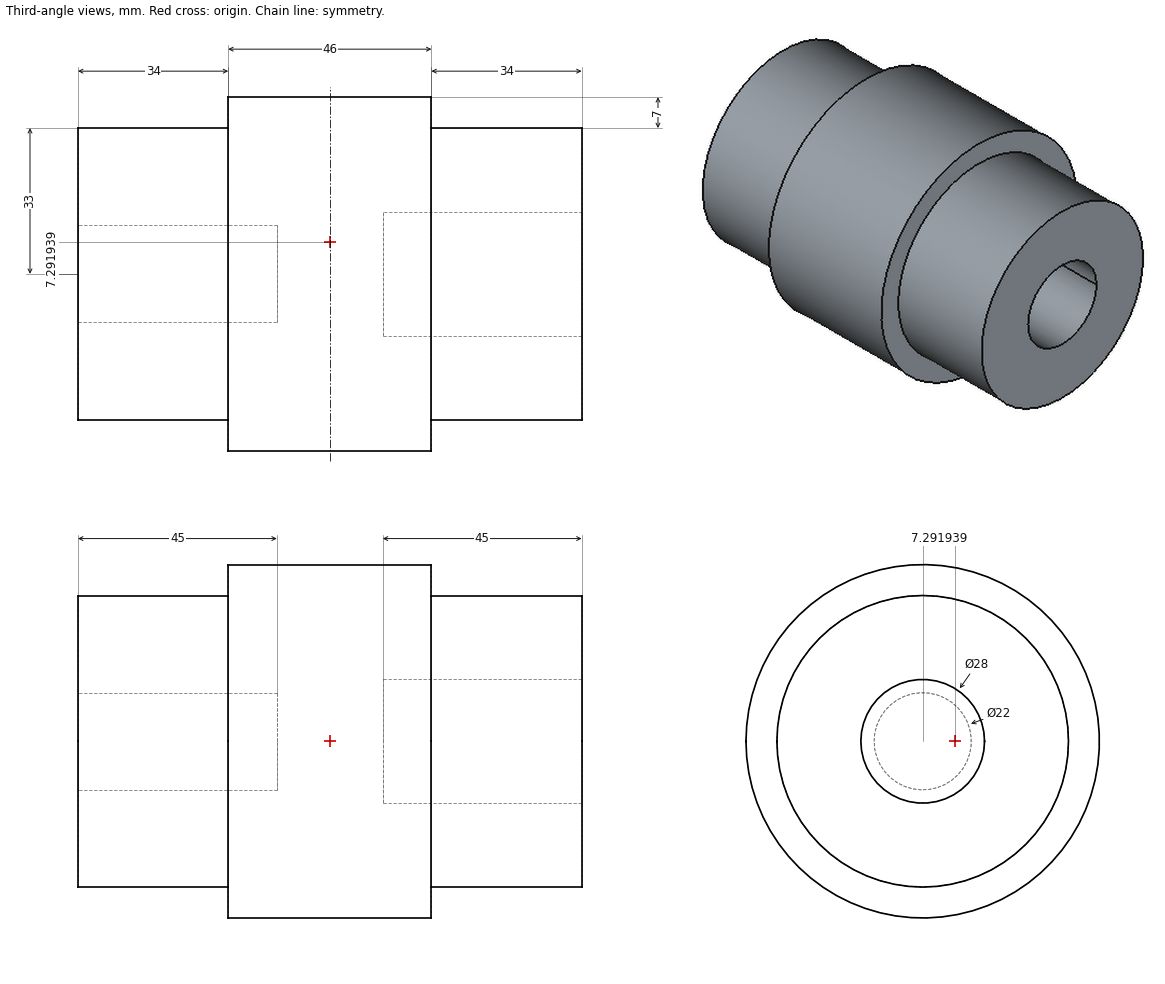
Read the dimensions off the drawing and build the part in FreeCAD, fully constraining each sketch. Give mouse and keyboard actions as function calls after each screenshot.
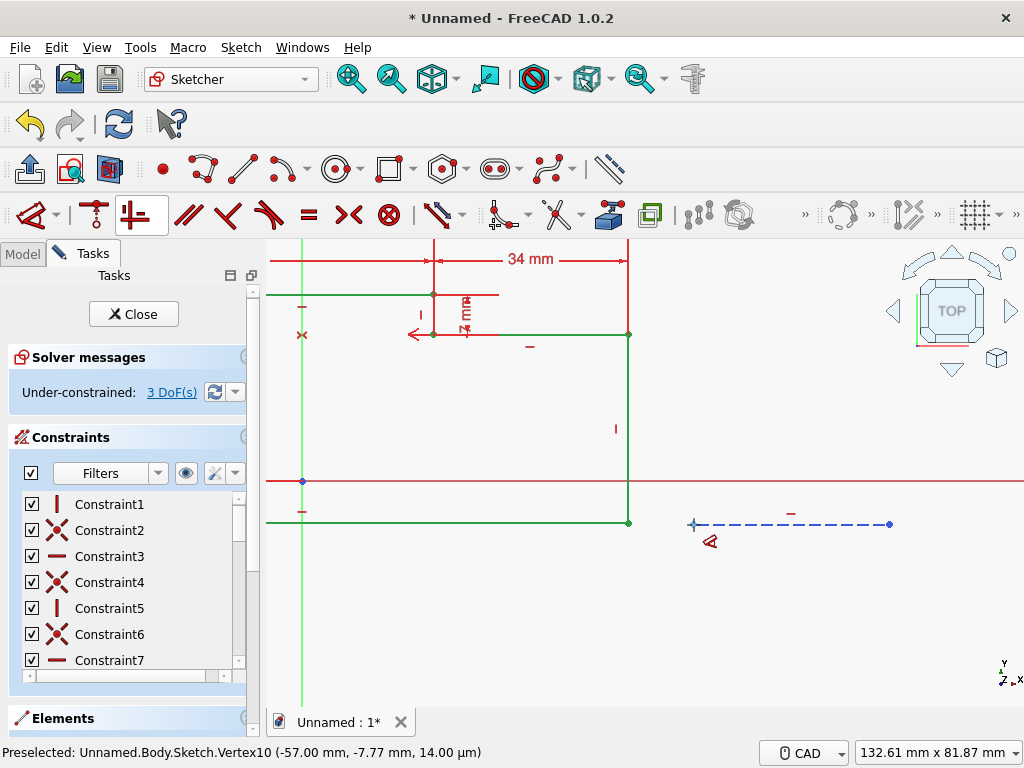
click(693, 525)
click(727, 503)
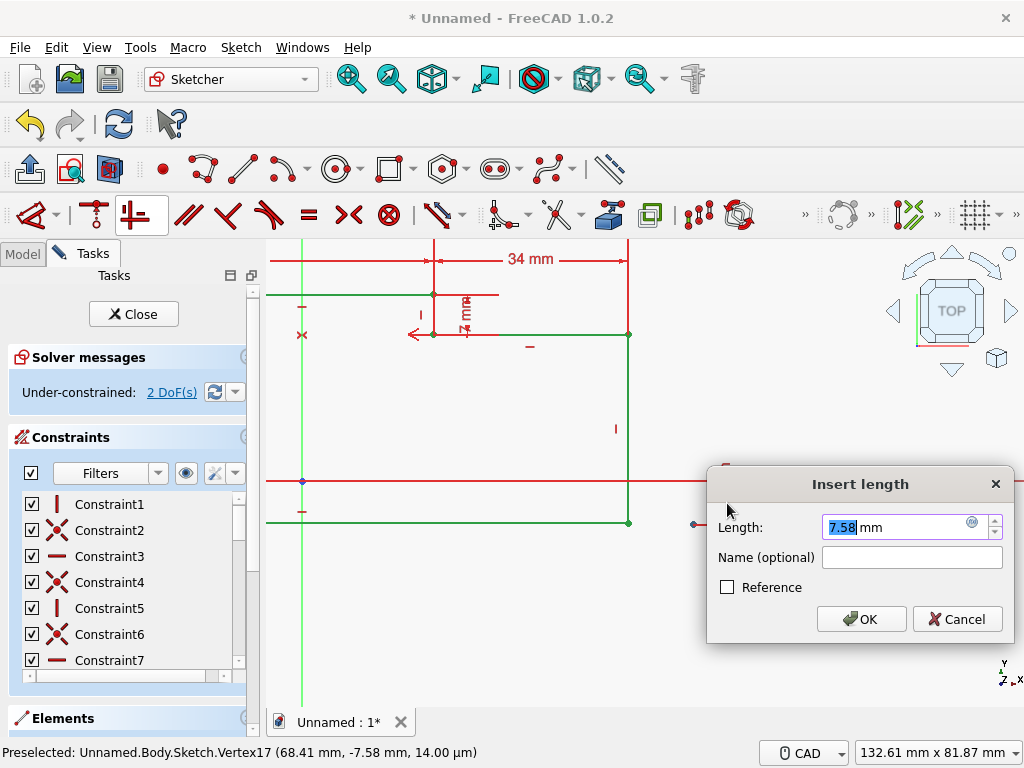
text(7.291939)
key(Return)
key(Escape)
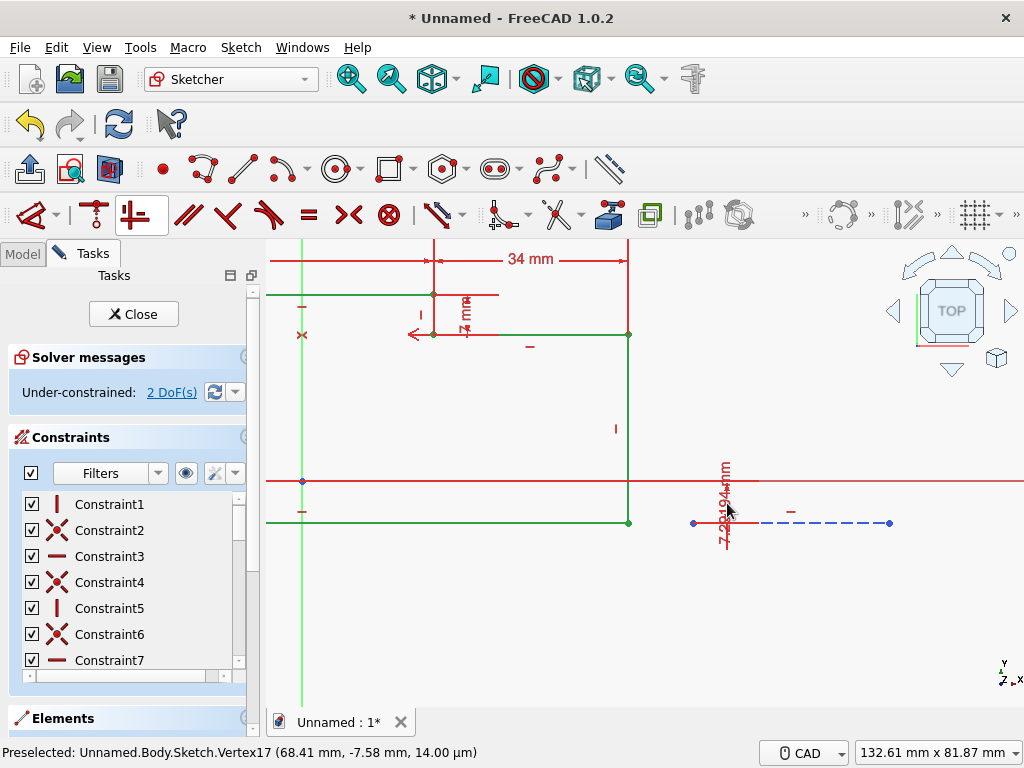
click(134, 314)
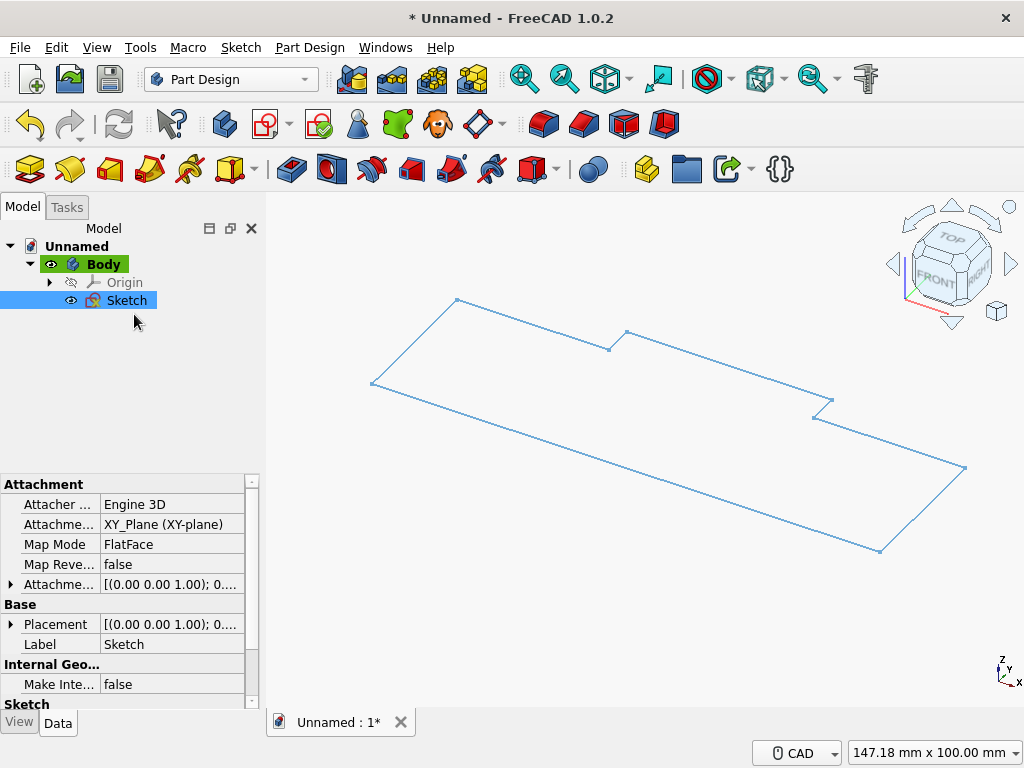
click(70, 170)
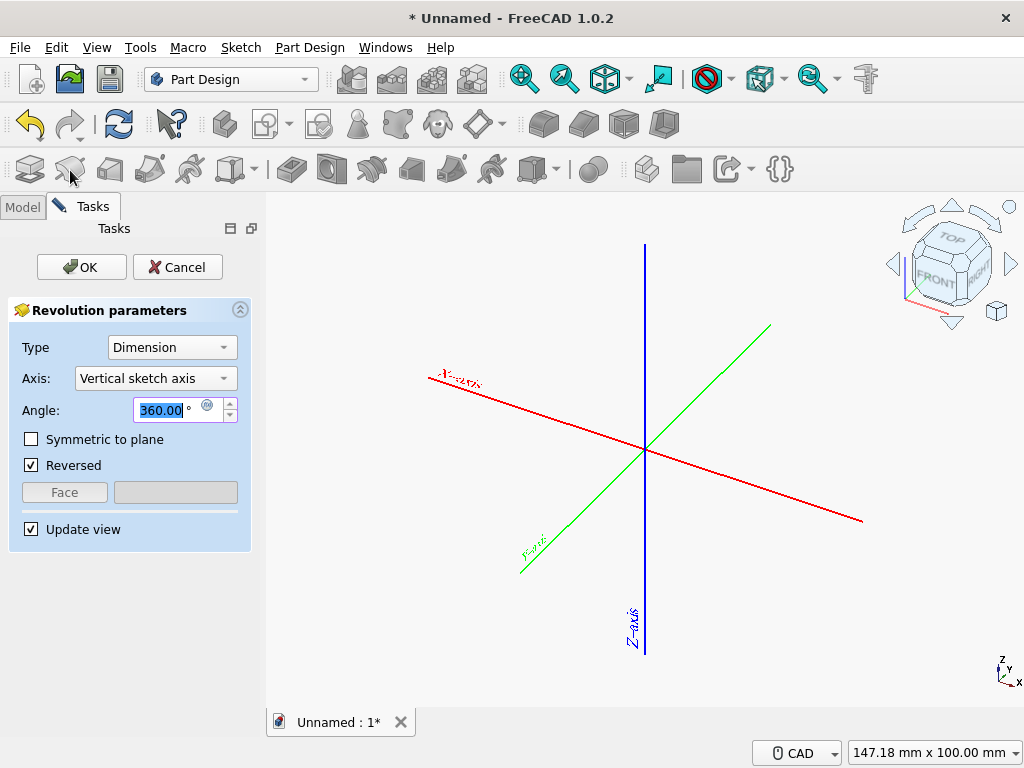
click(156, 378)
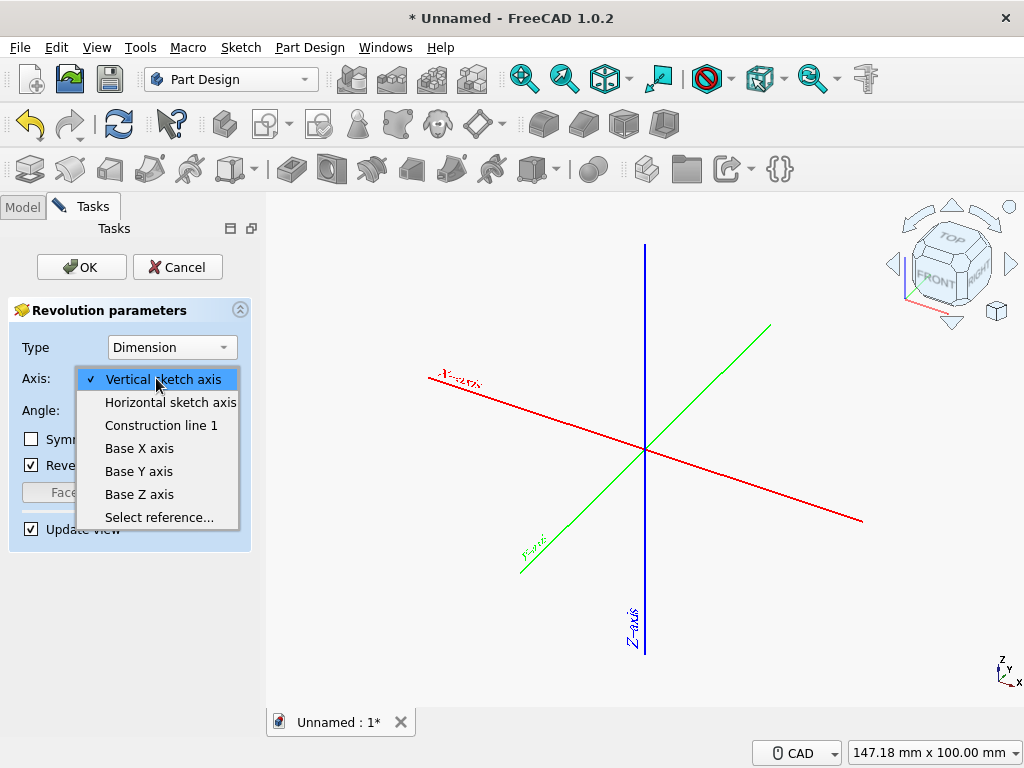
click(156, 426)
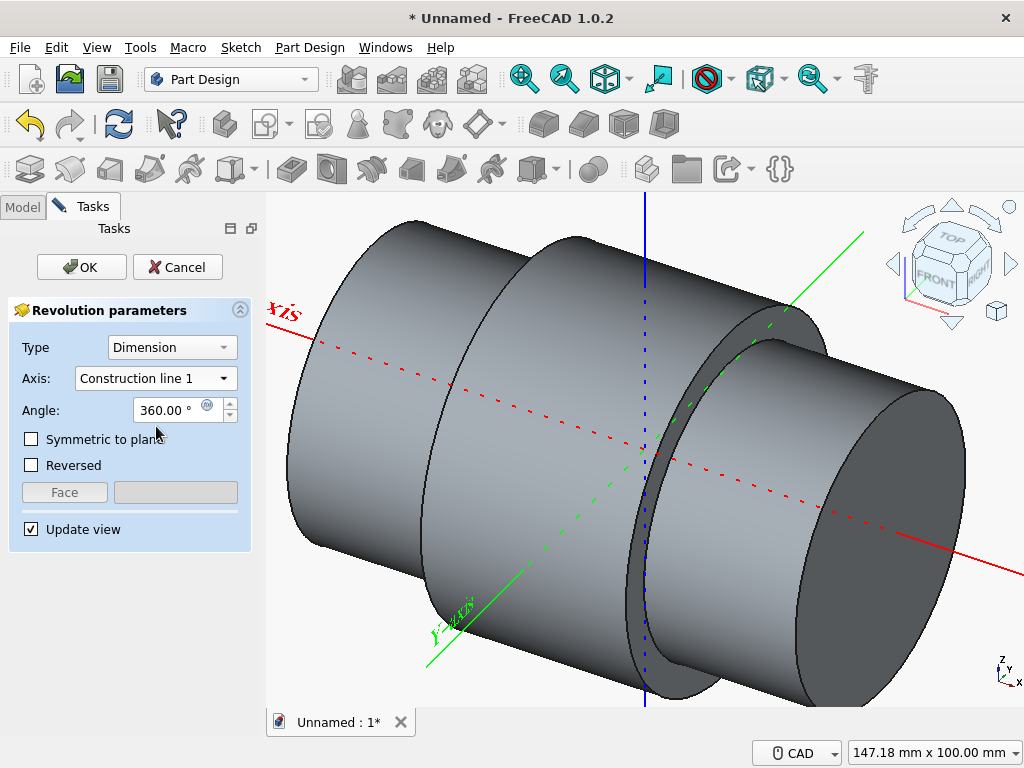
click(82, 267)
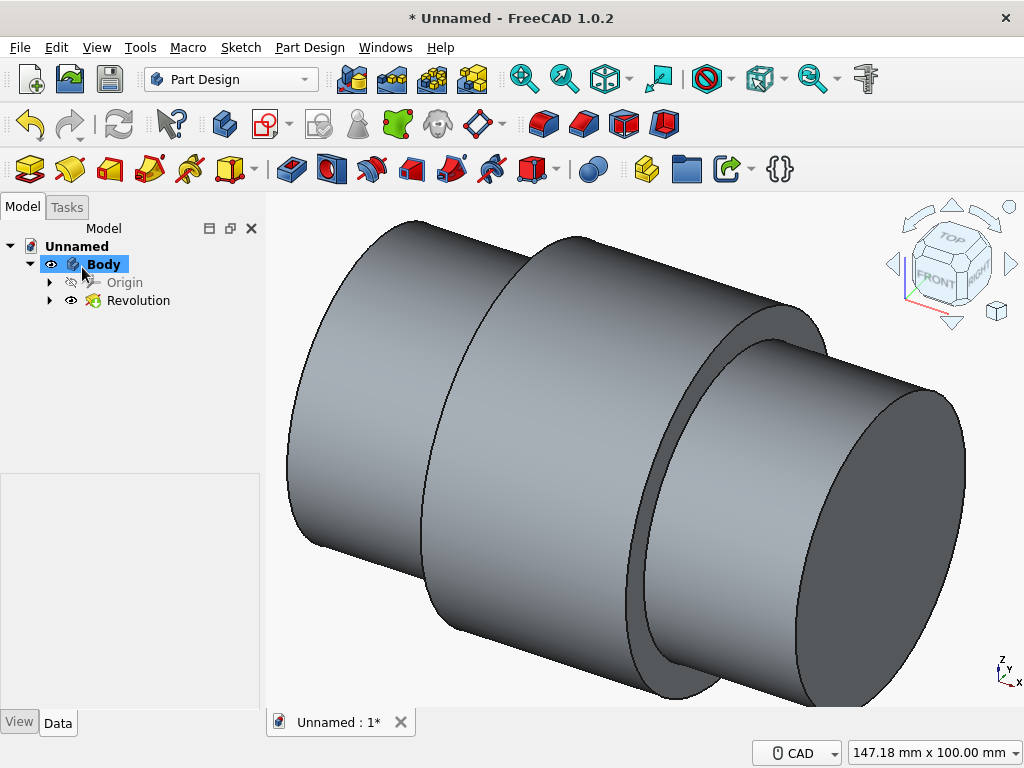
click(526, 80)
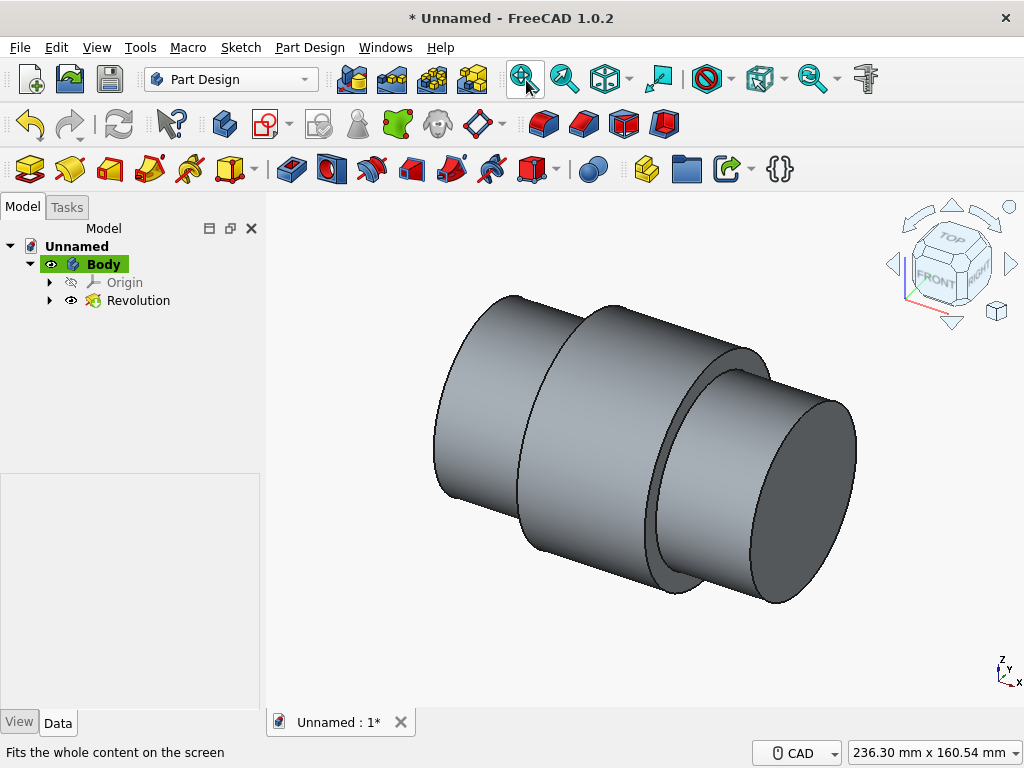
key(6)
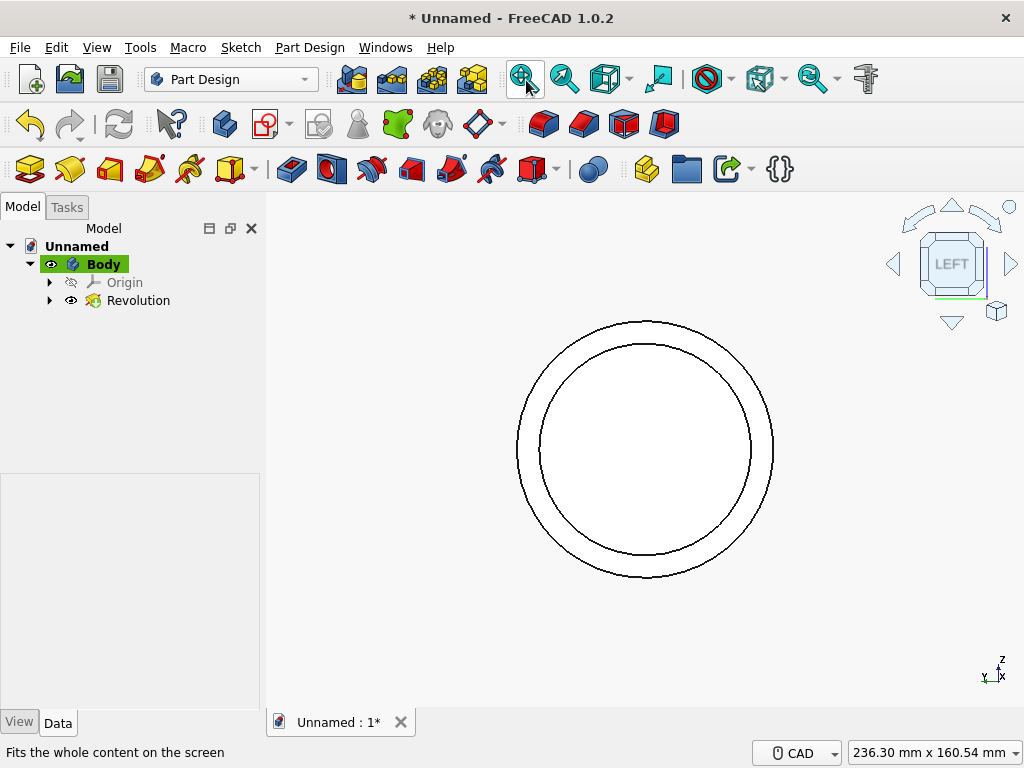
click(645, 448)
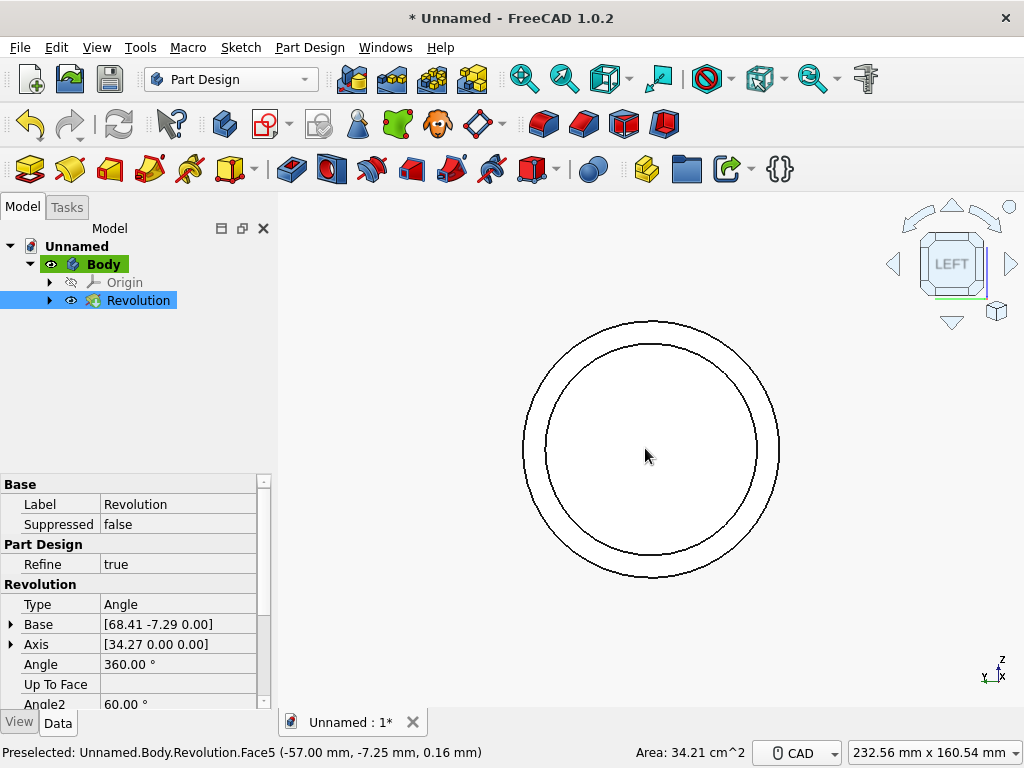
click(266, 124)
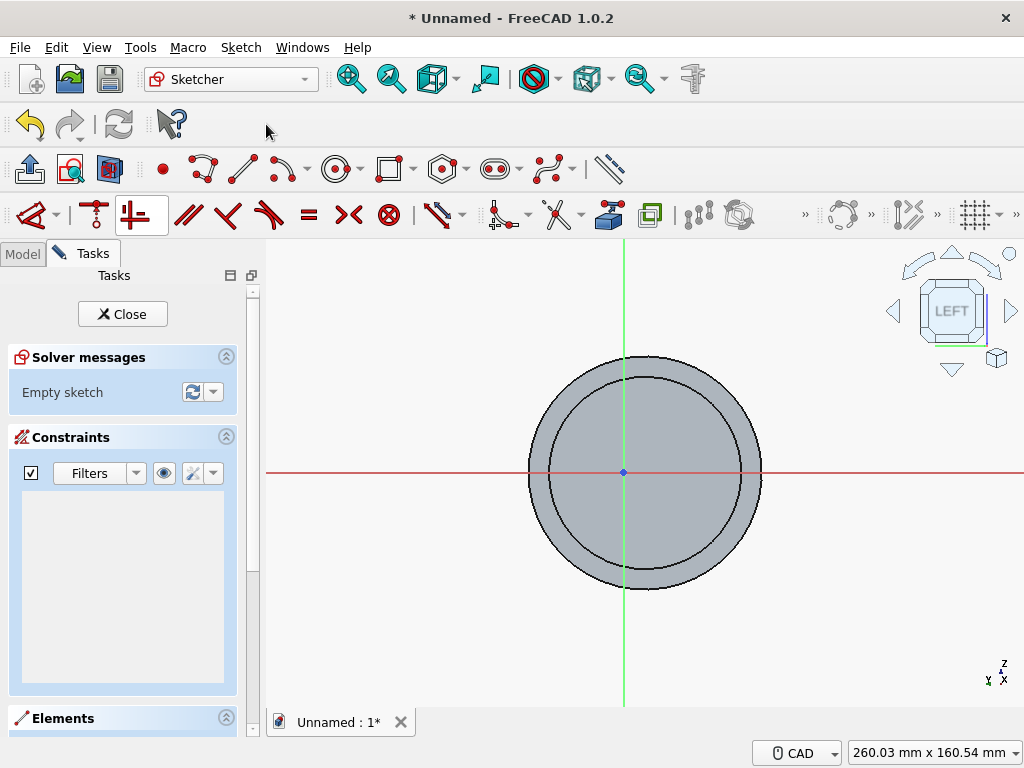
scroll(662, 473, up, 8)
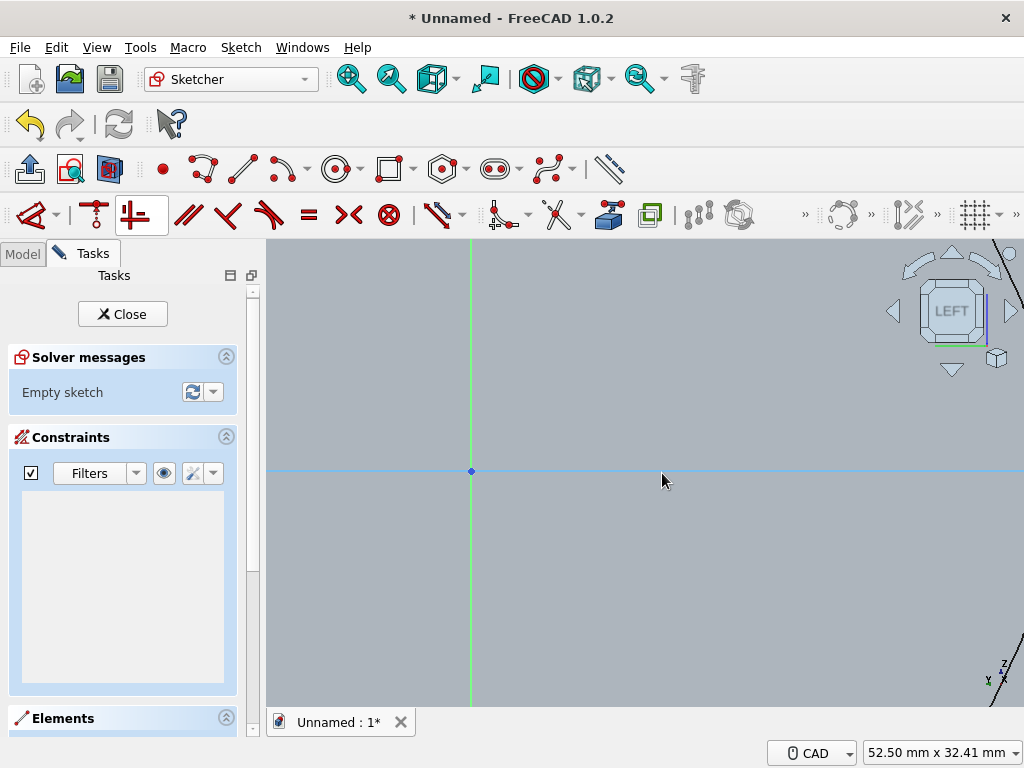
click(336, 170)